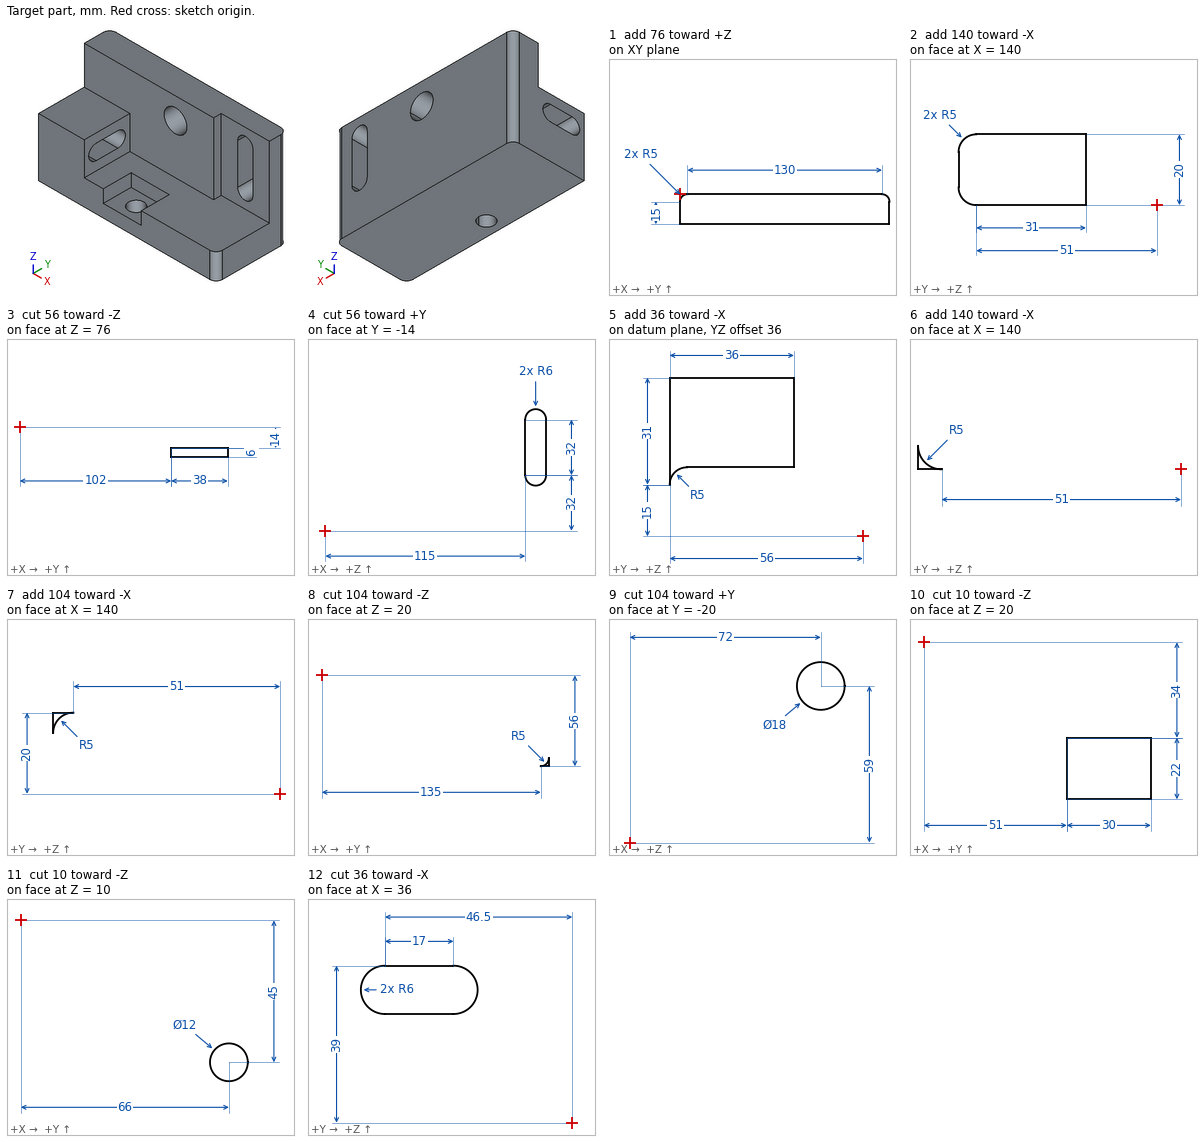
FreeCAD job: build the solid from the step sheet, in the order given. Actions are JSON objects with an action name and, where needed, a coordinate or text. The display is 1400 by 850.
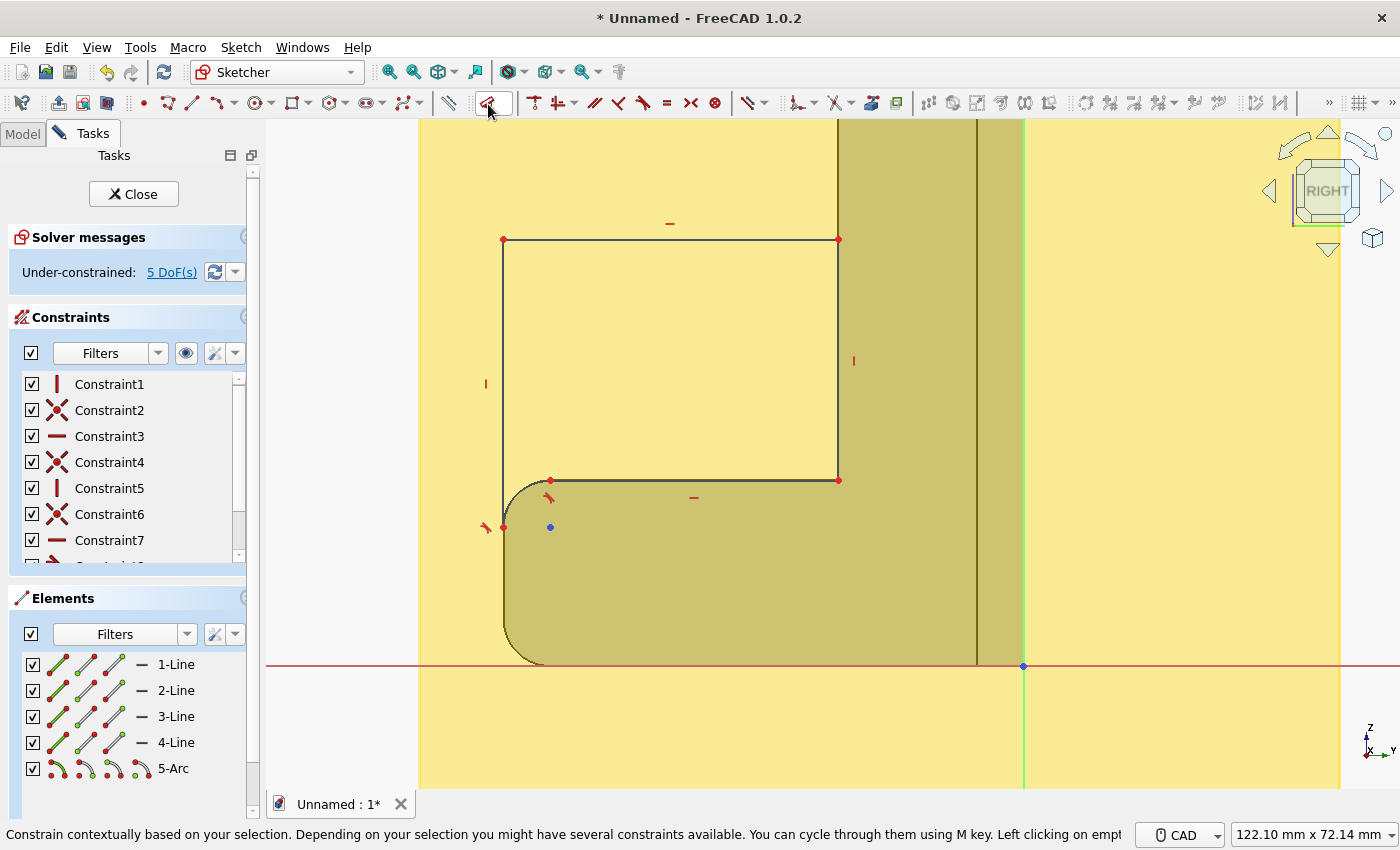
{"action": "left_click", "coordinate": [529, 486]}
{"action": "left_click", "coordinate": [553, 449]}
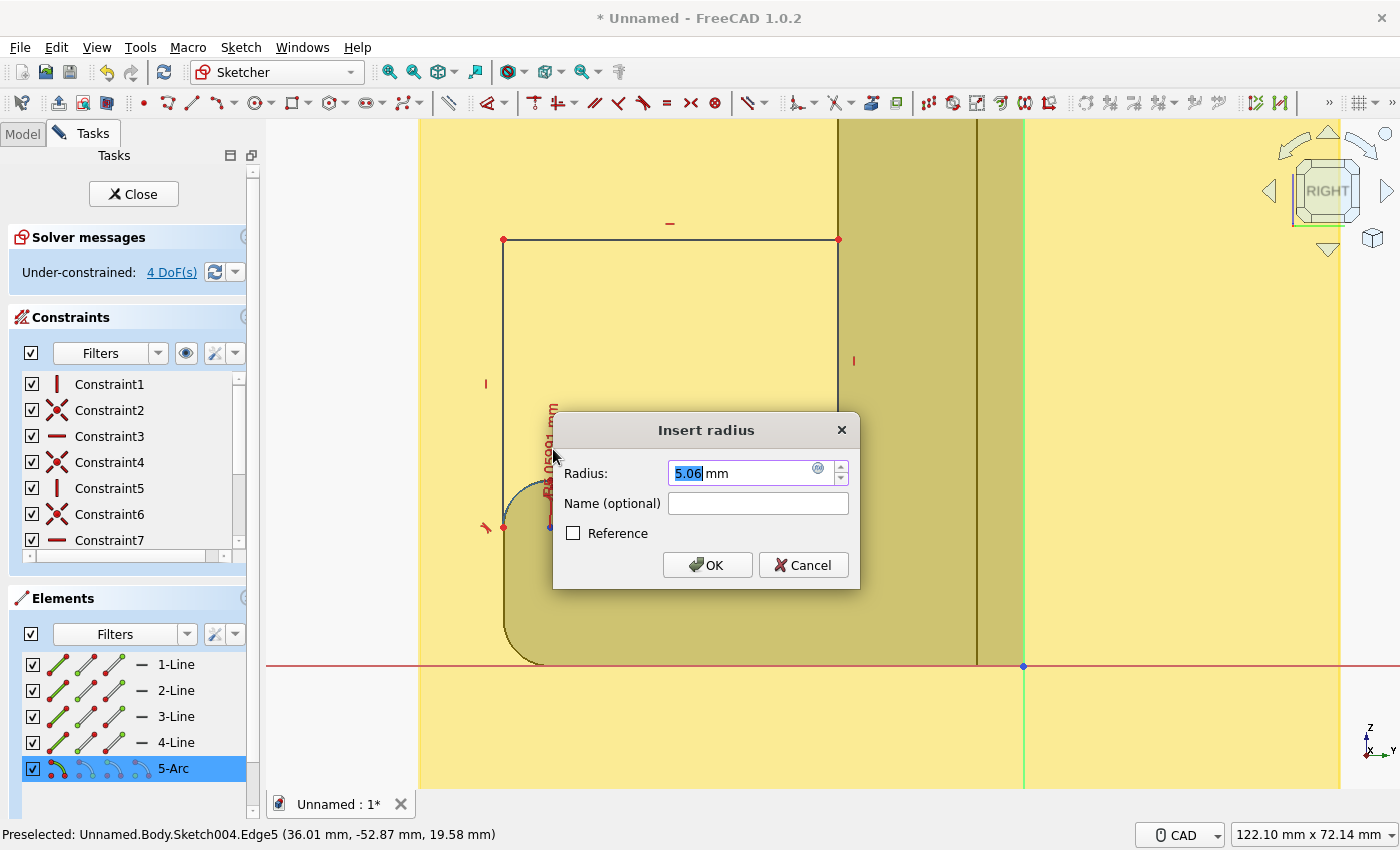
{"action": "type", "text": "5"}
{"action": "key", "text": "Return"}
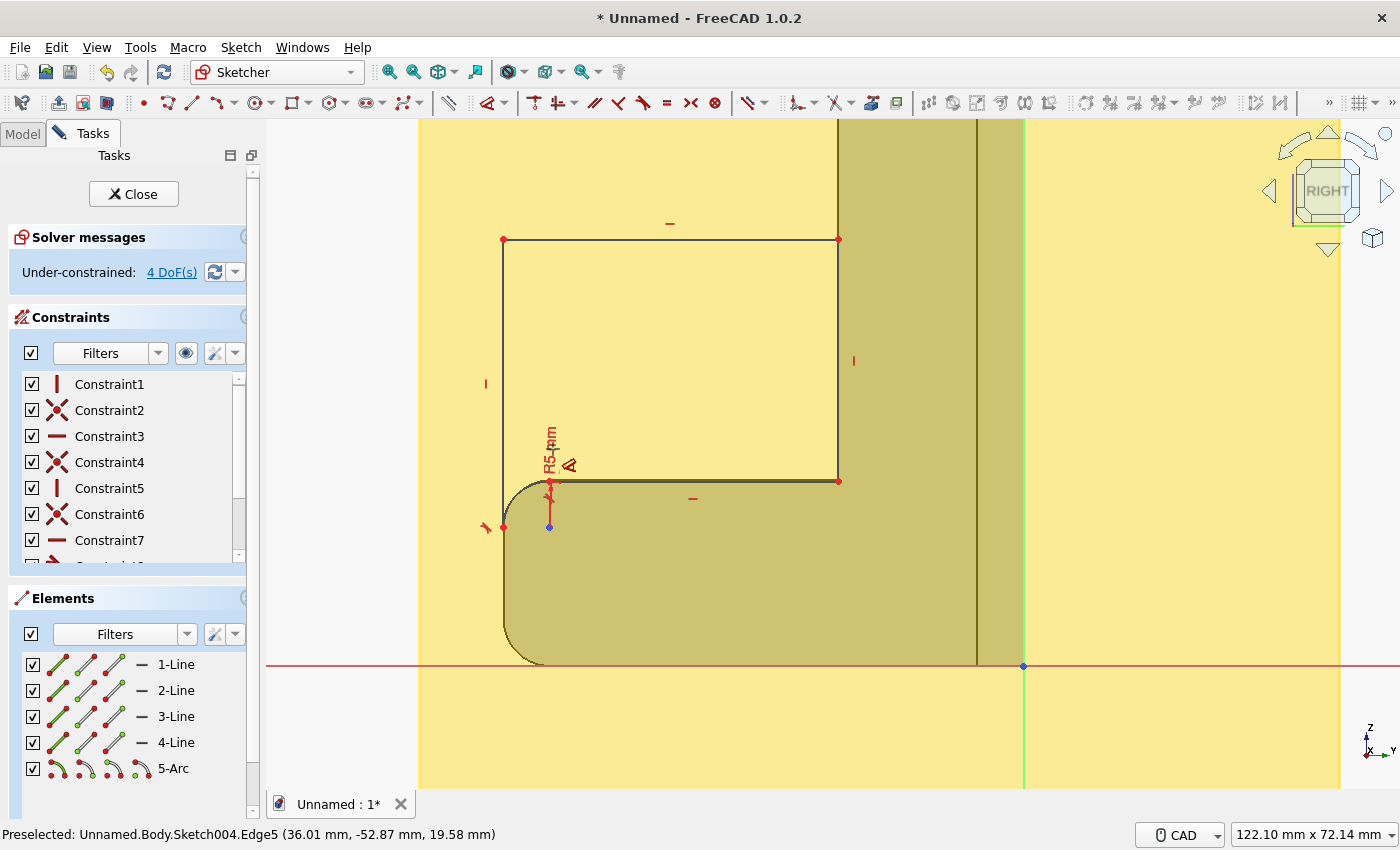
{"action": "left_click", "coordinate": [503, 442]}
{"action": "left_click", "coordinate": [469, 384]}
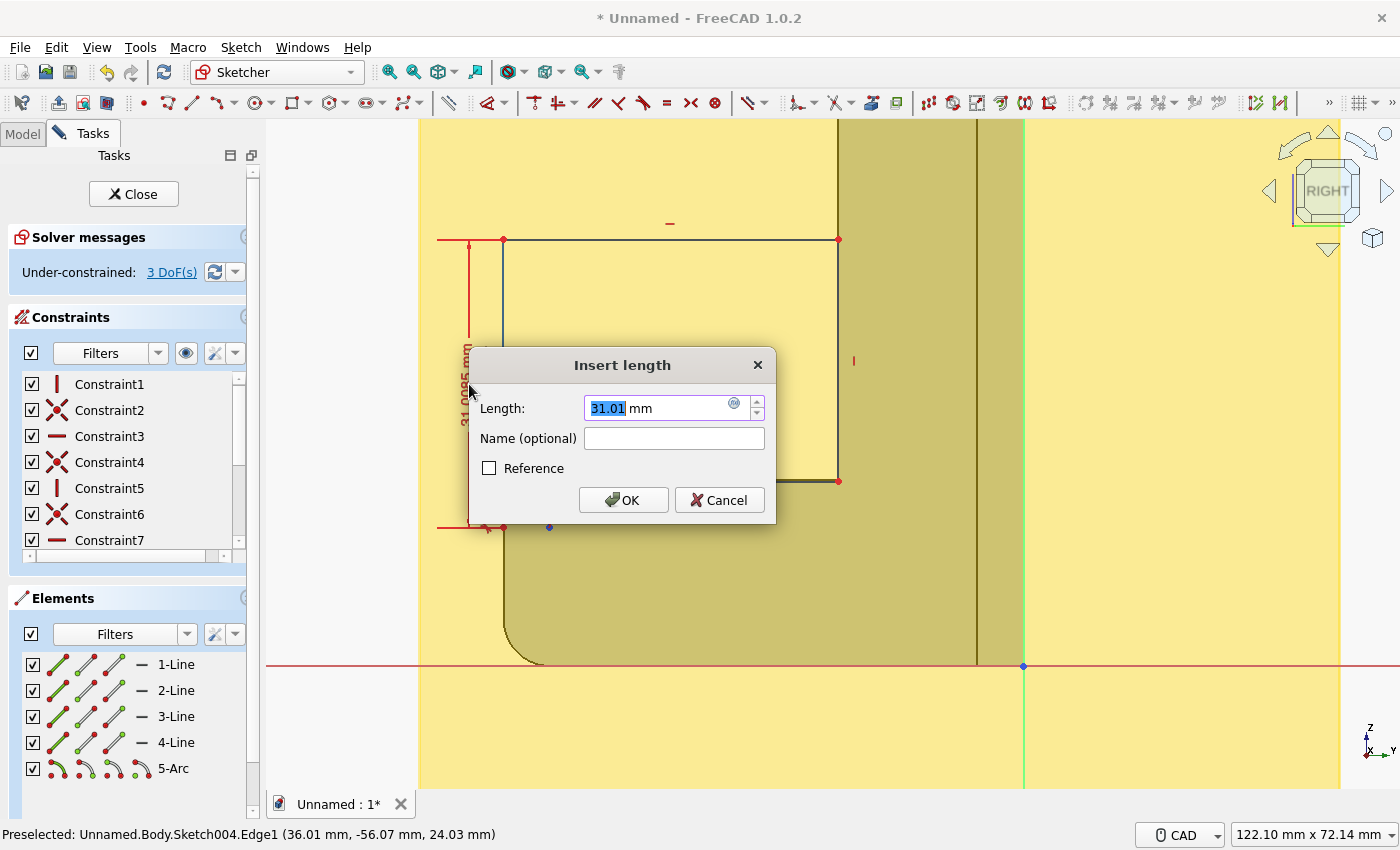
{"action": "type", "text": "31"}
{"action": "key", "text": "Return"}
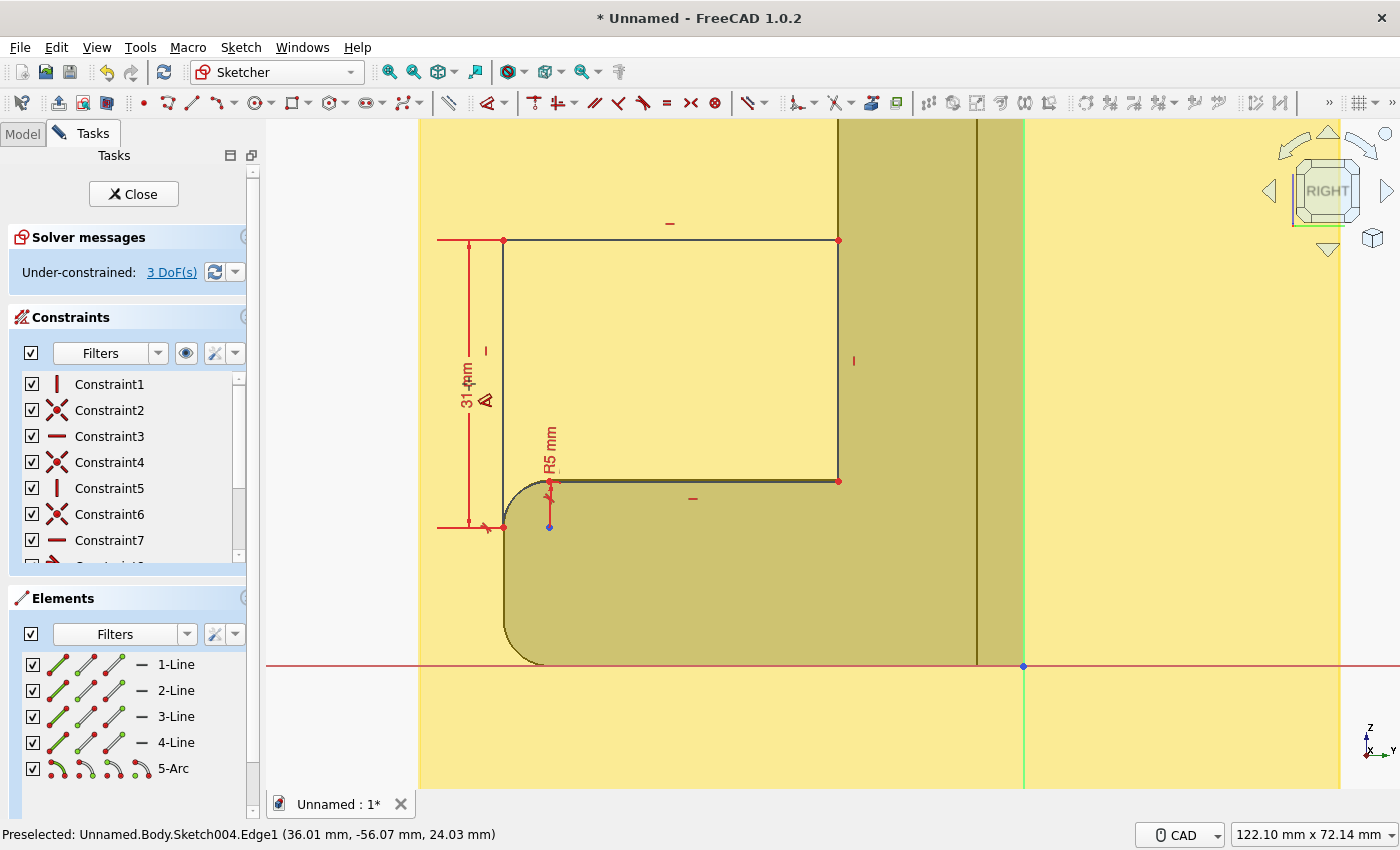
{"action": "left_click", "coordinate": [604, 240]}
{"action": "left_click", "coordinate": [671, 206]}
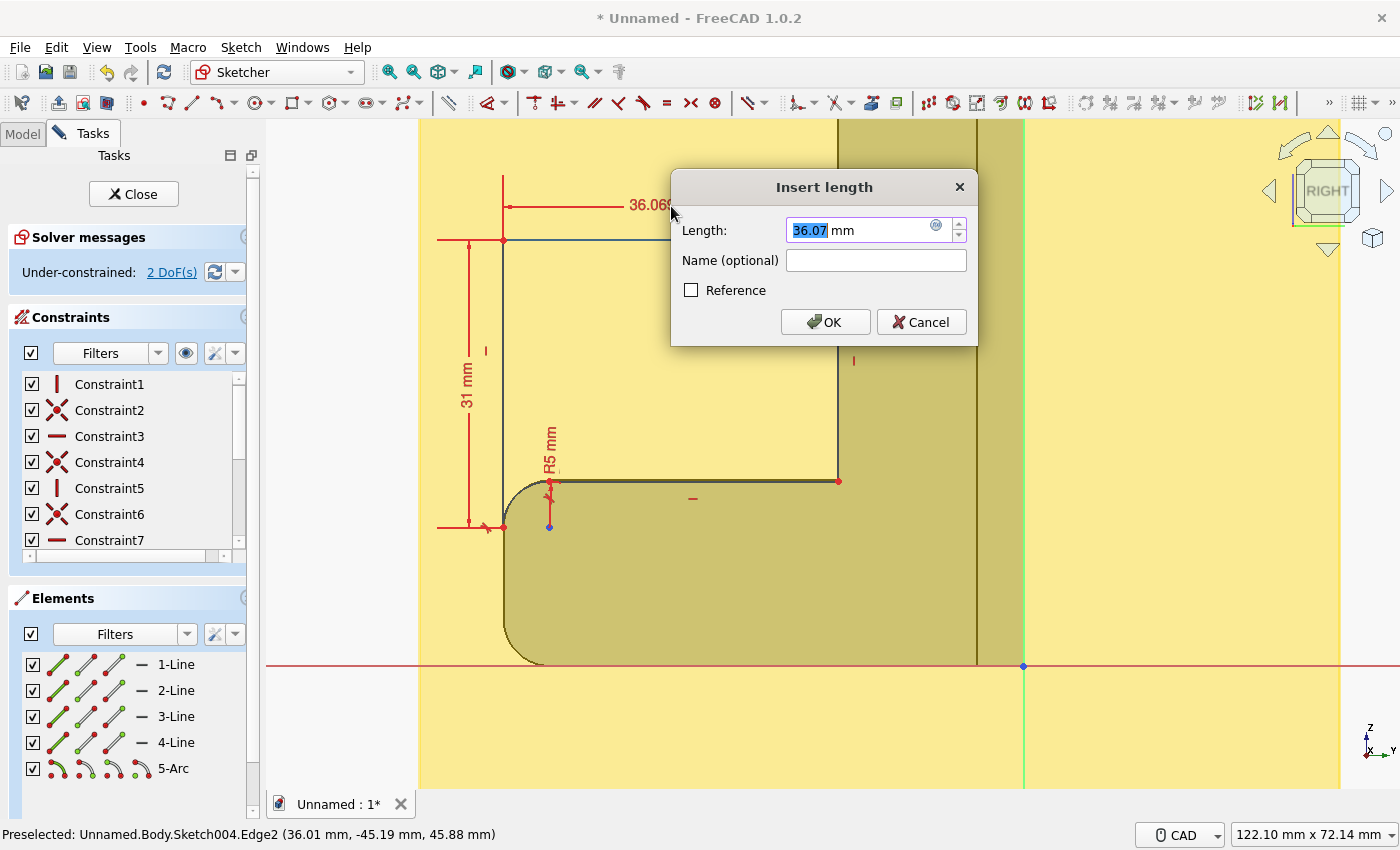
{"action": "type", "text": "36"}
{"action": "key", "text": "Return"}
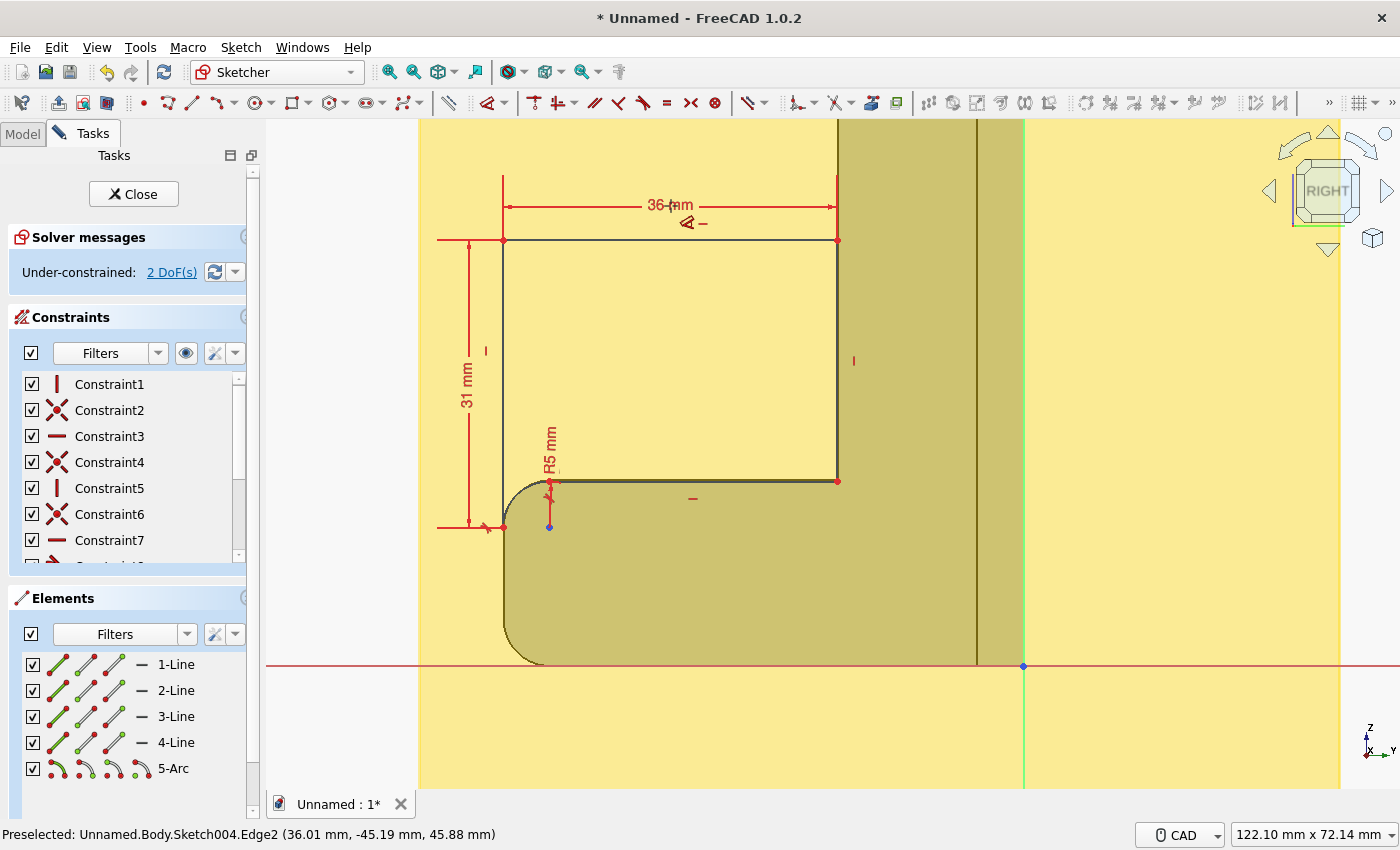
{"action": "left_click", "coordinate": [503, 528]}
{"action": "left_click", "coordinate": [763, 700]}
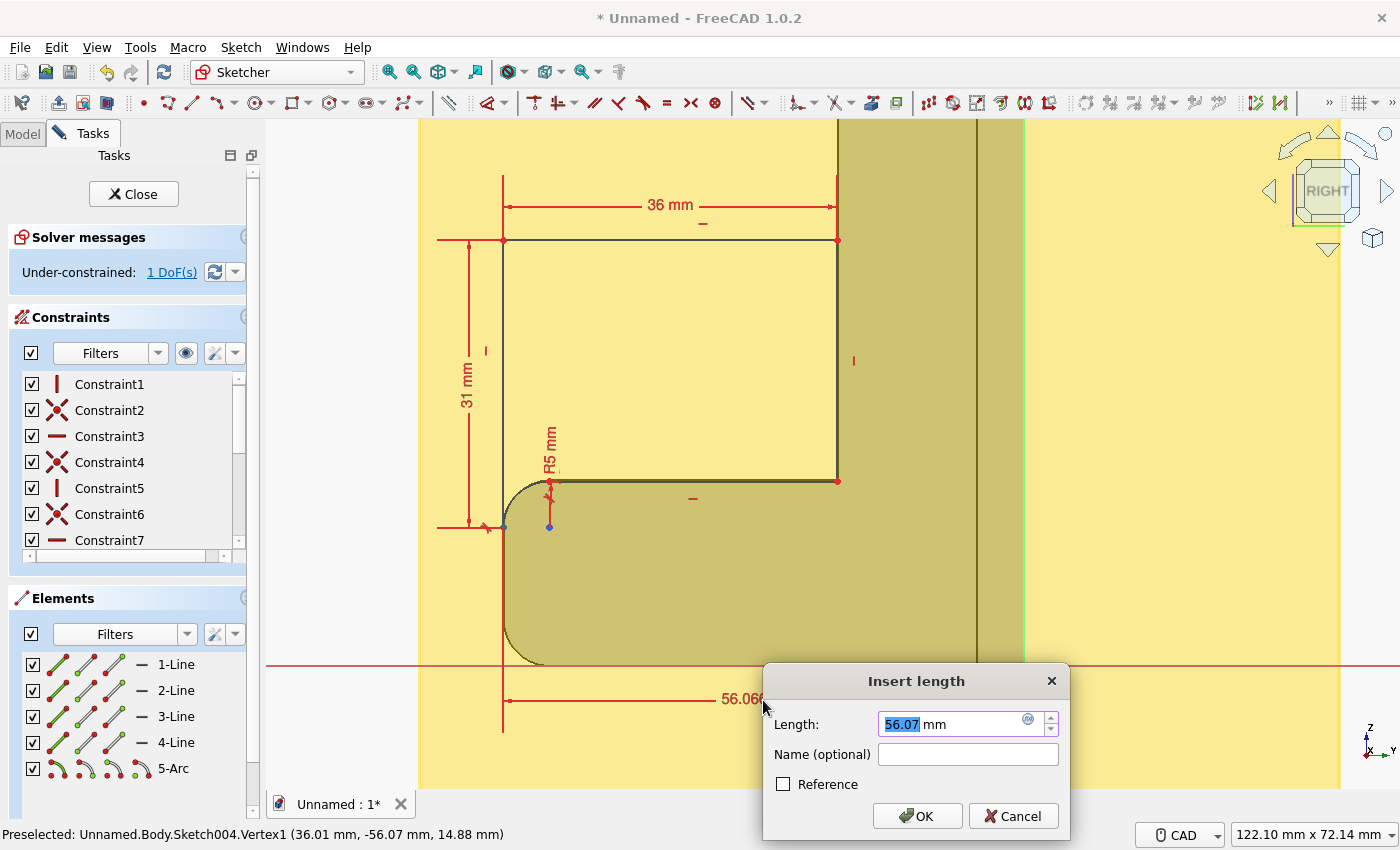
{"action": "type", "text": "56"}
{"action": "key", "text": "Return"}